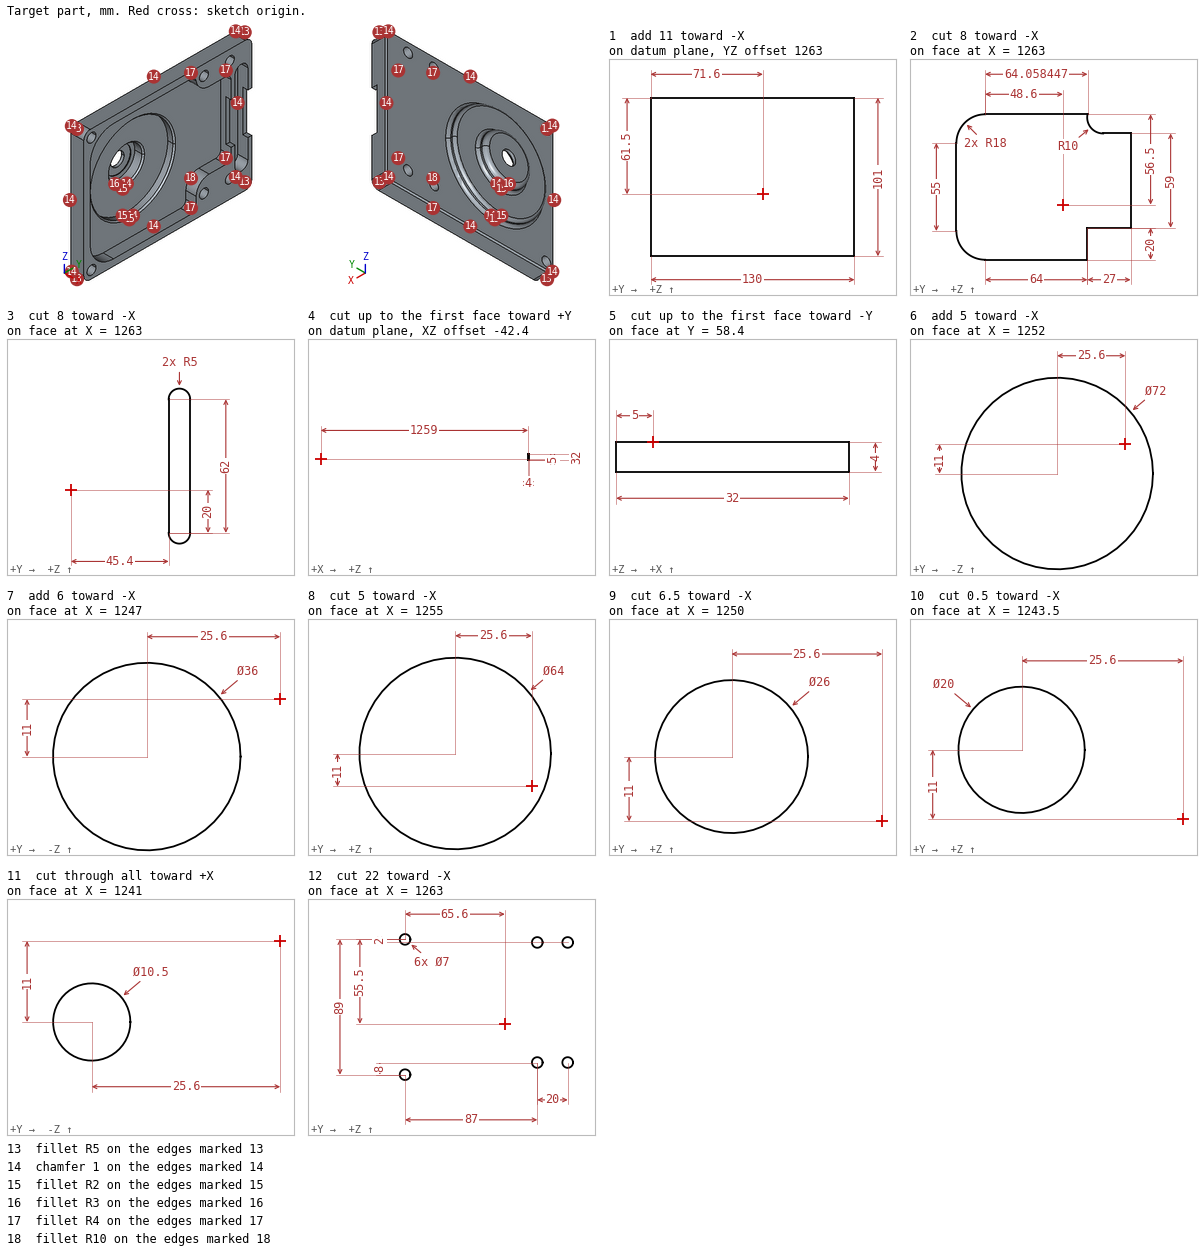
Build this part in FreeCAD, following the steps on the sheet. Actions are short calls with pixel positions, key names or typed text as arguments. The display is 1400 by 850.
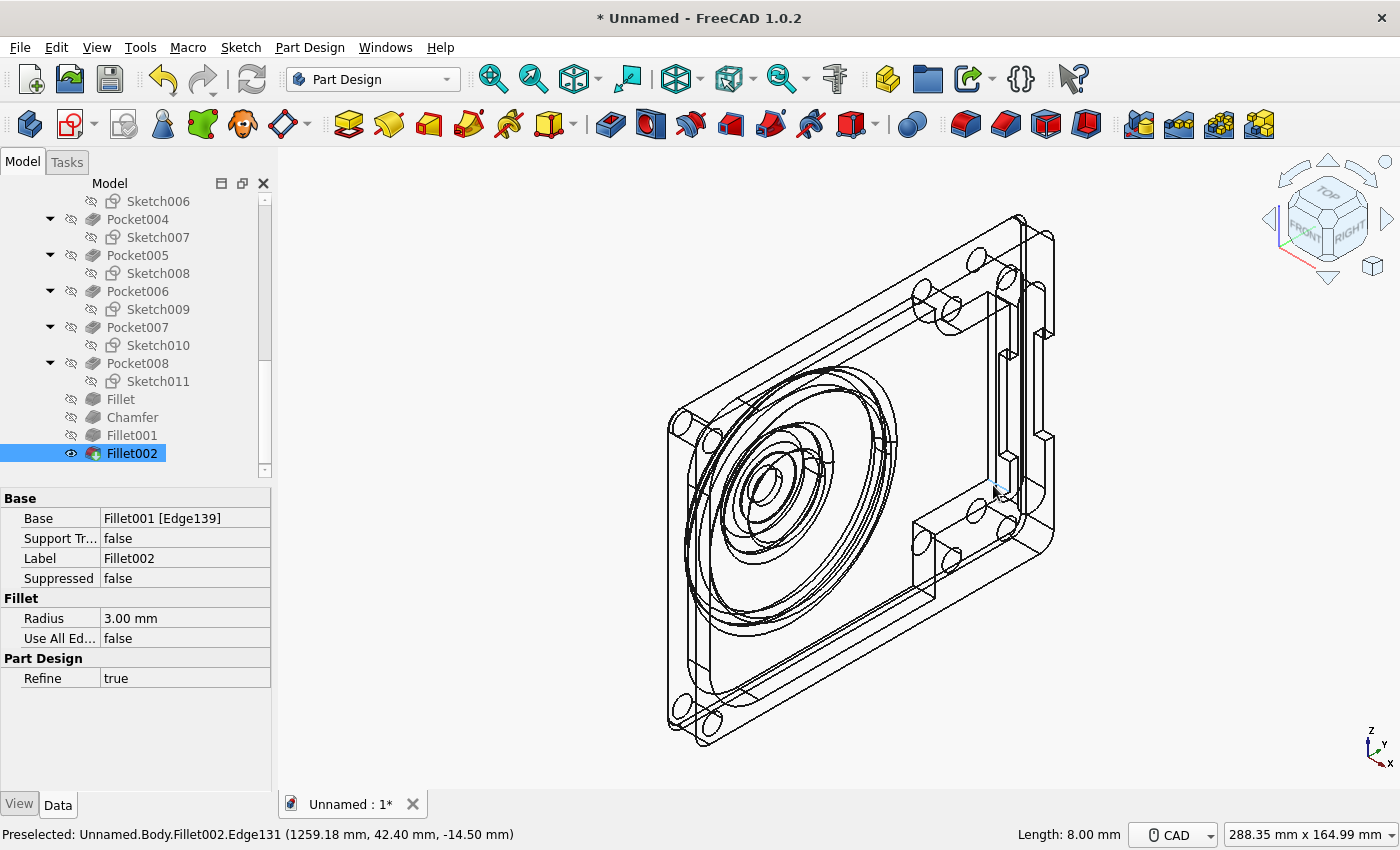
click(924, 591, ctrl)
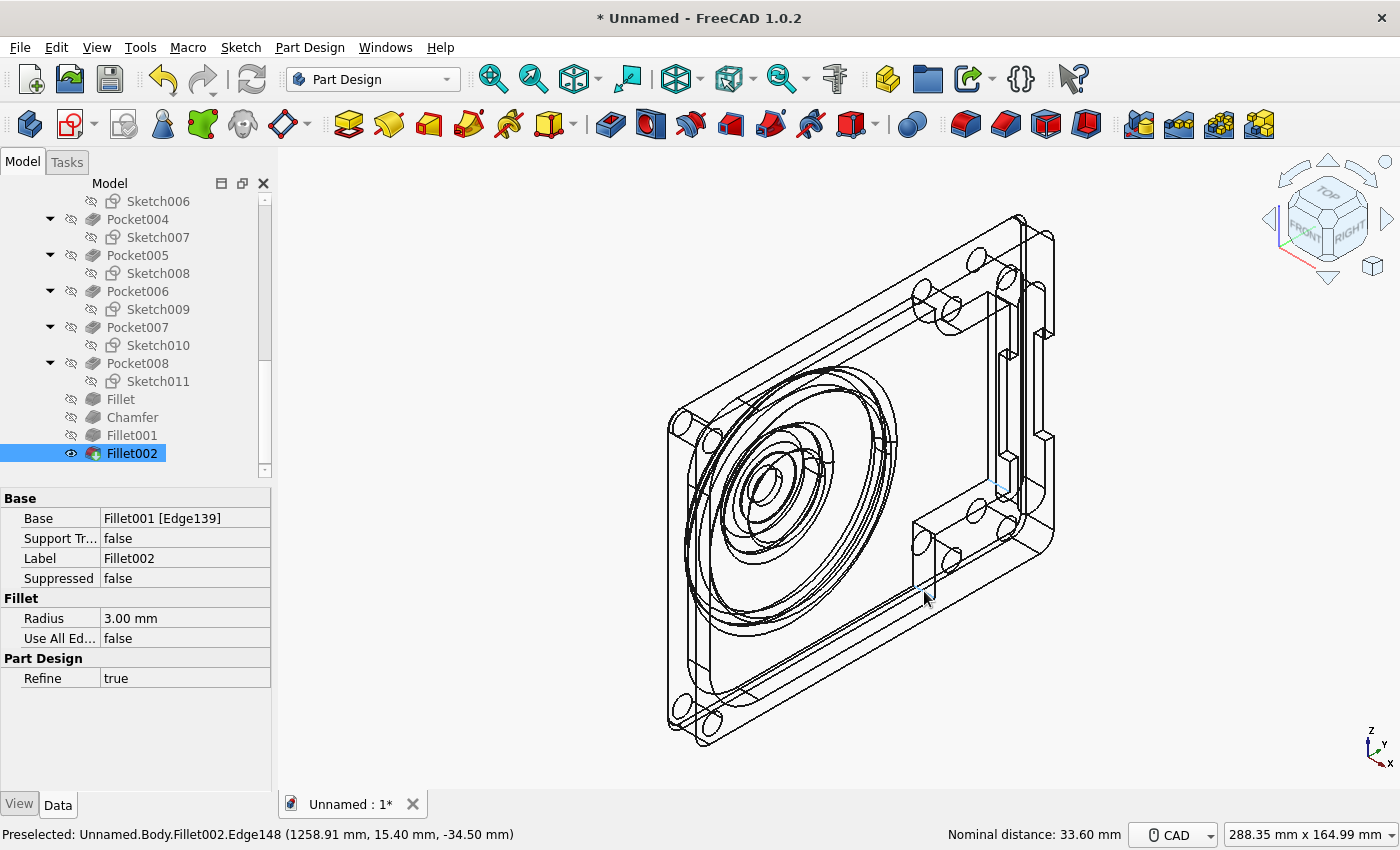
click(929, 304, ctrl)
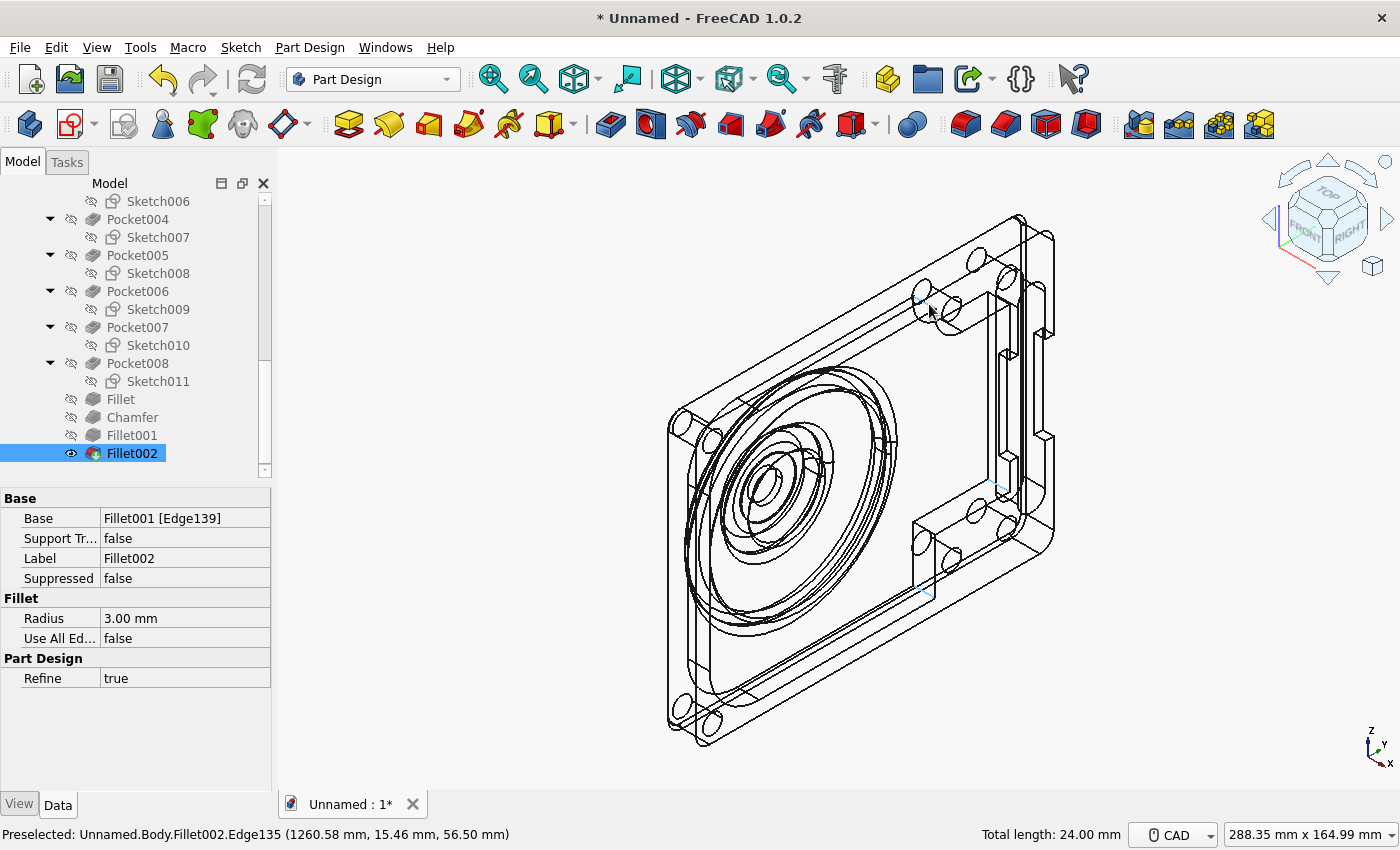
click(999, 297, ctrl)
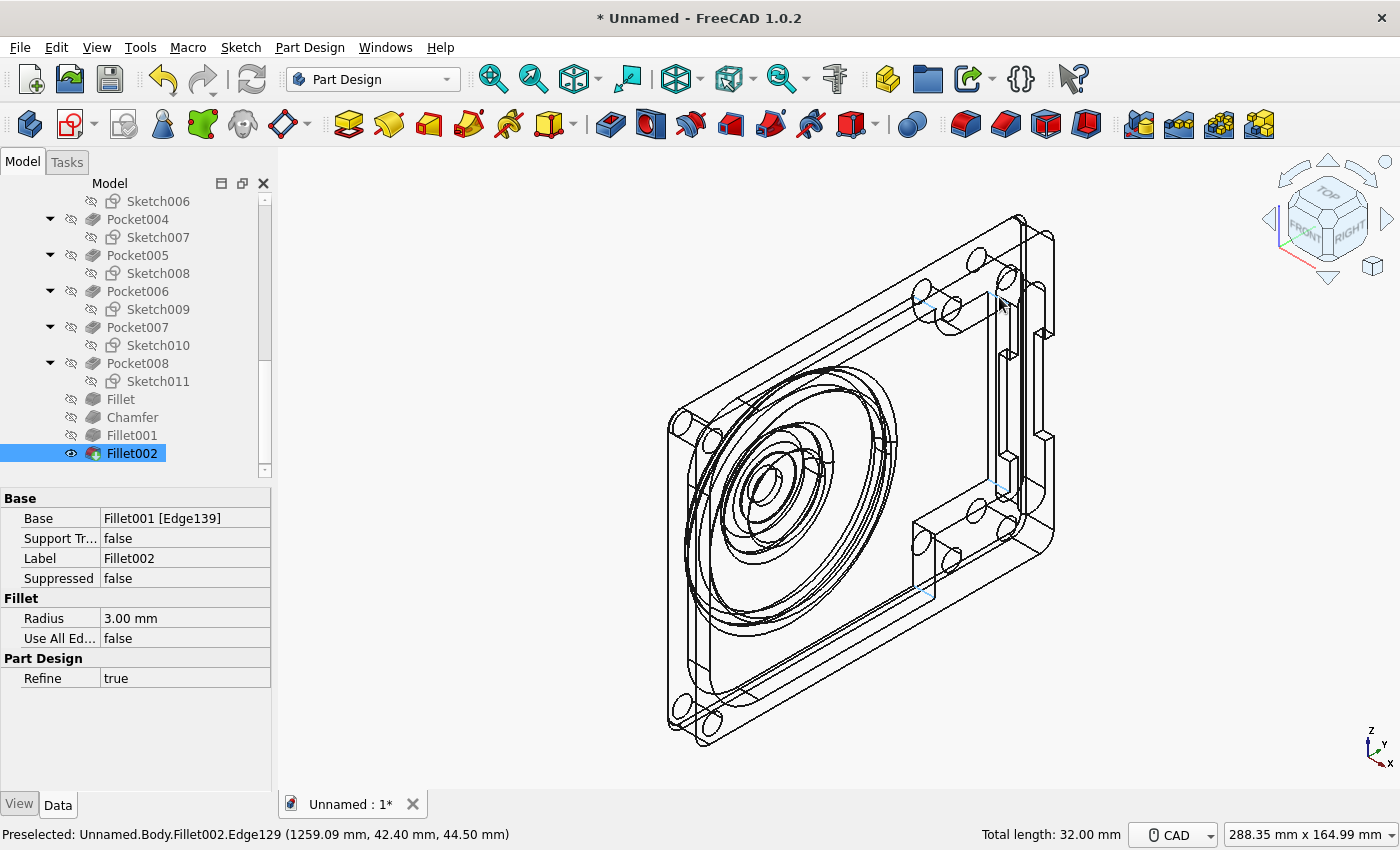
key(v)
key(1)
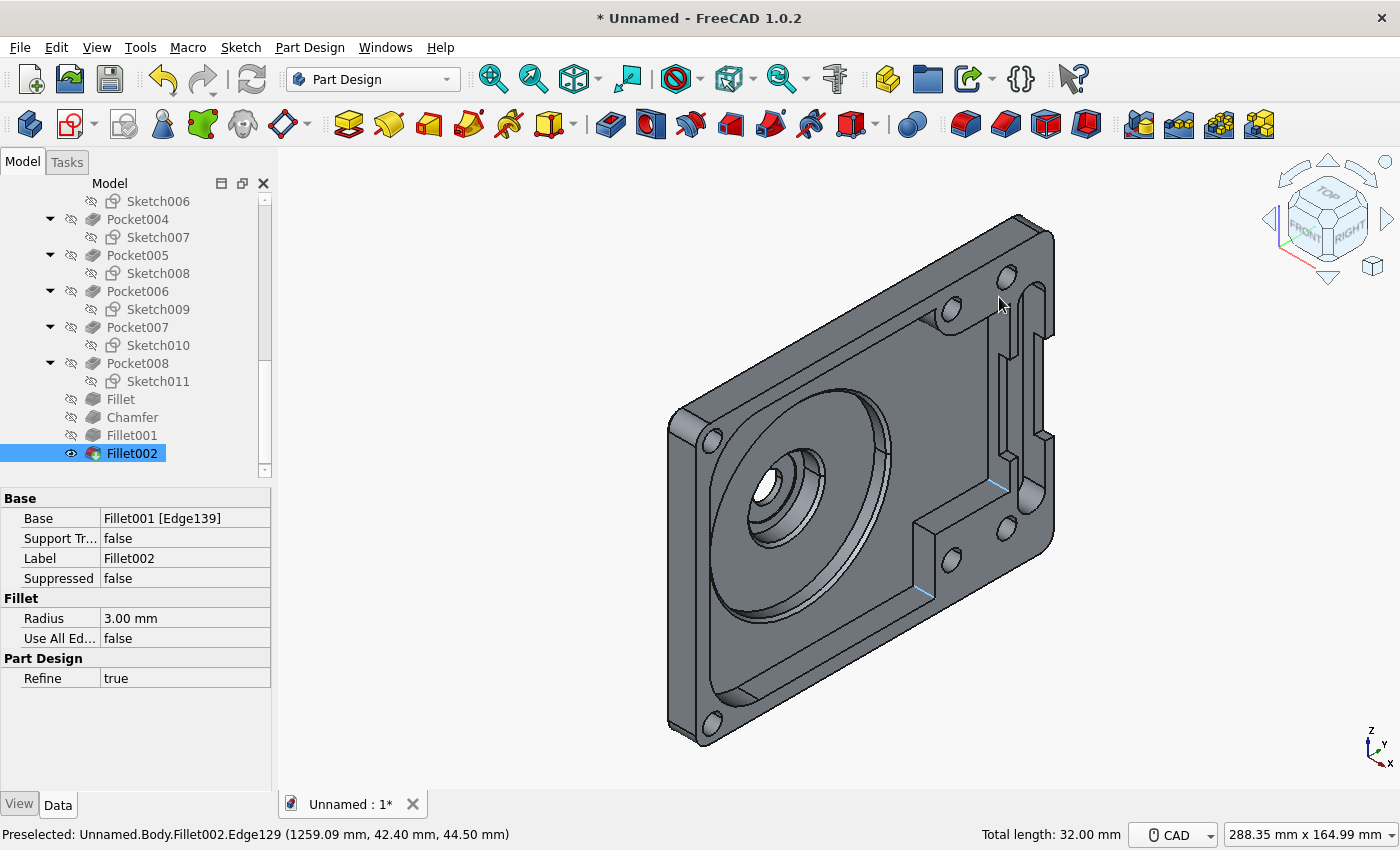
click(966, 124)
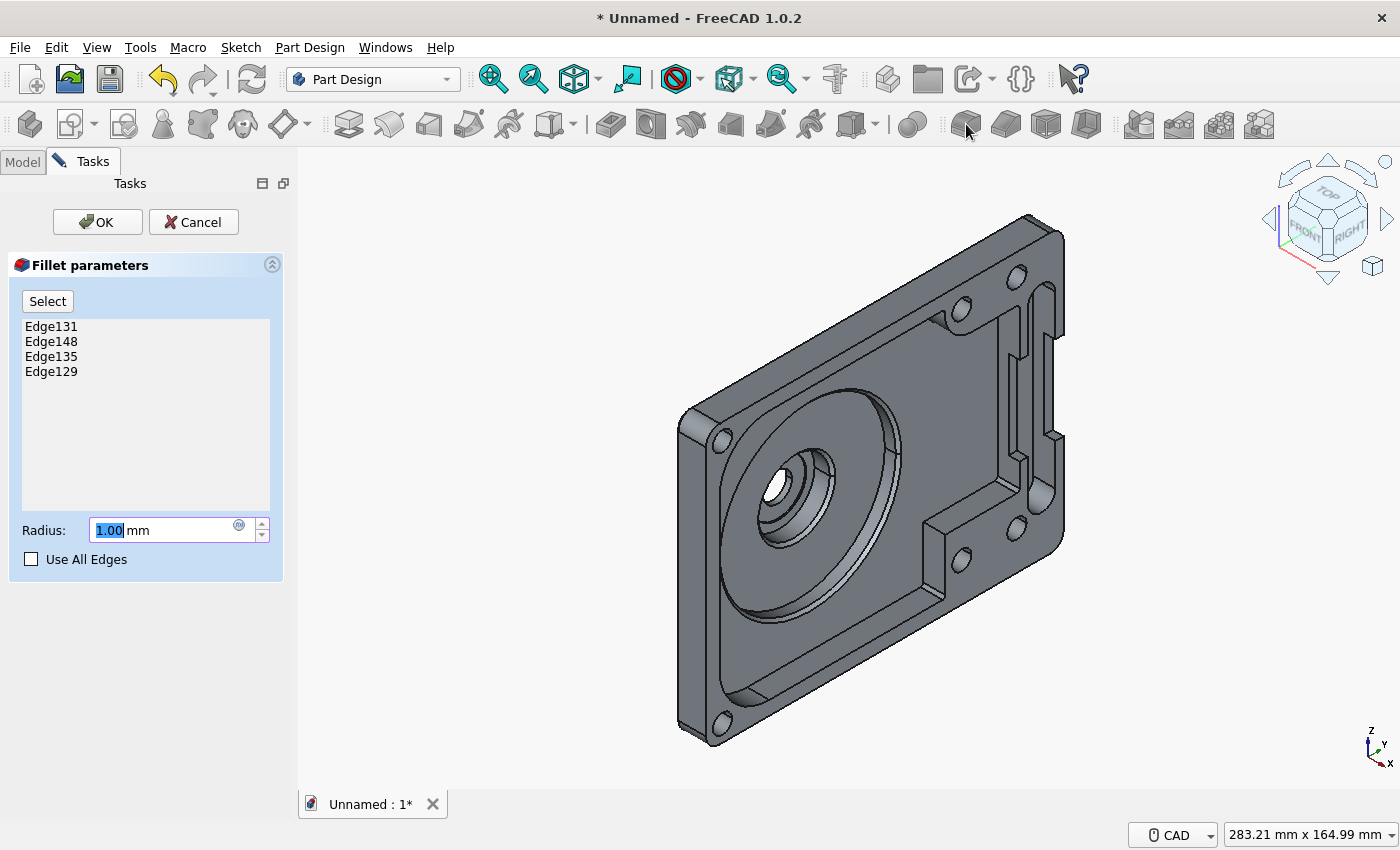
text(4)
key(Tab)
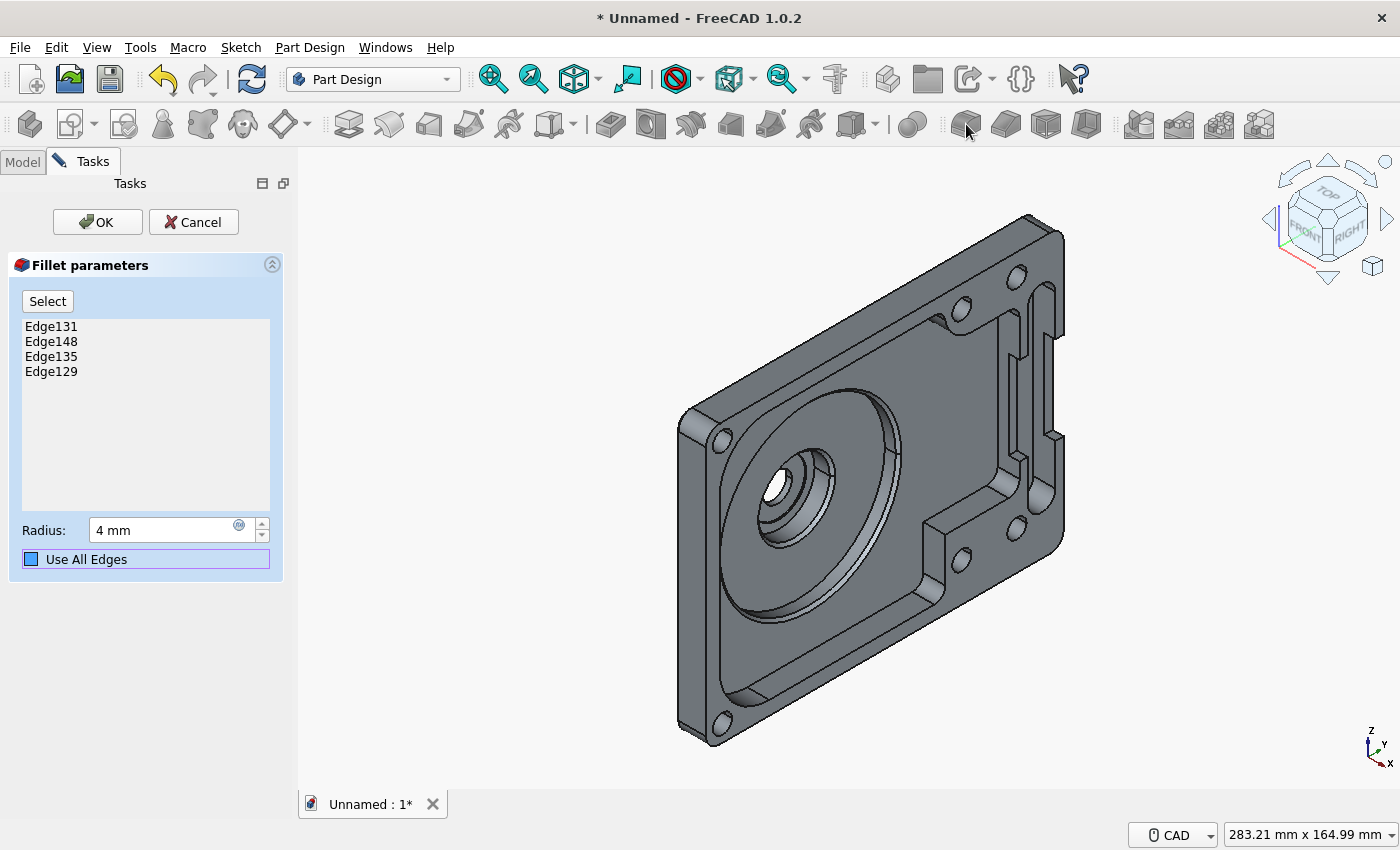
click(98, 222)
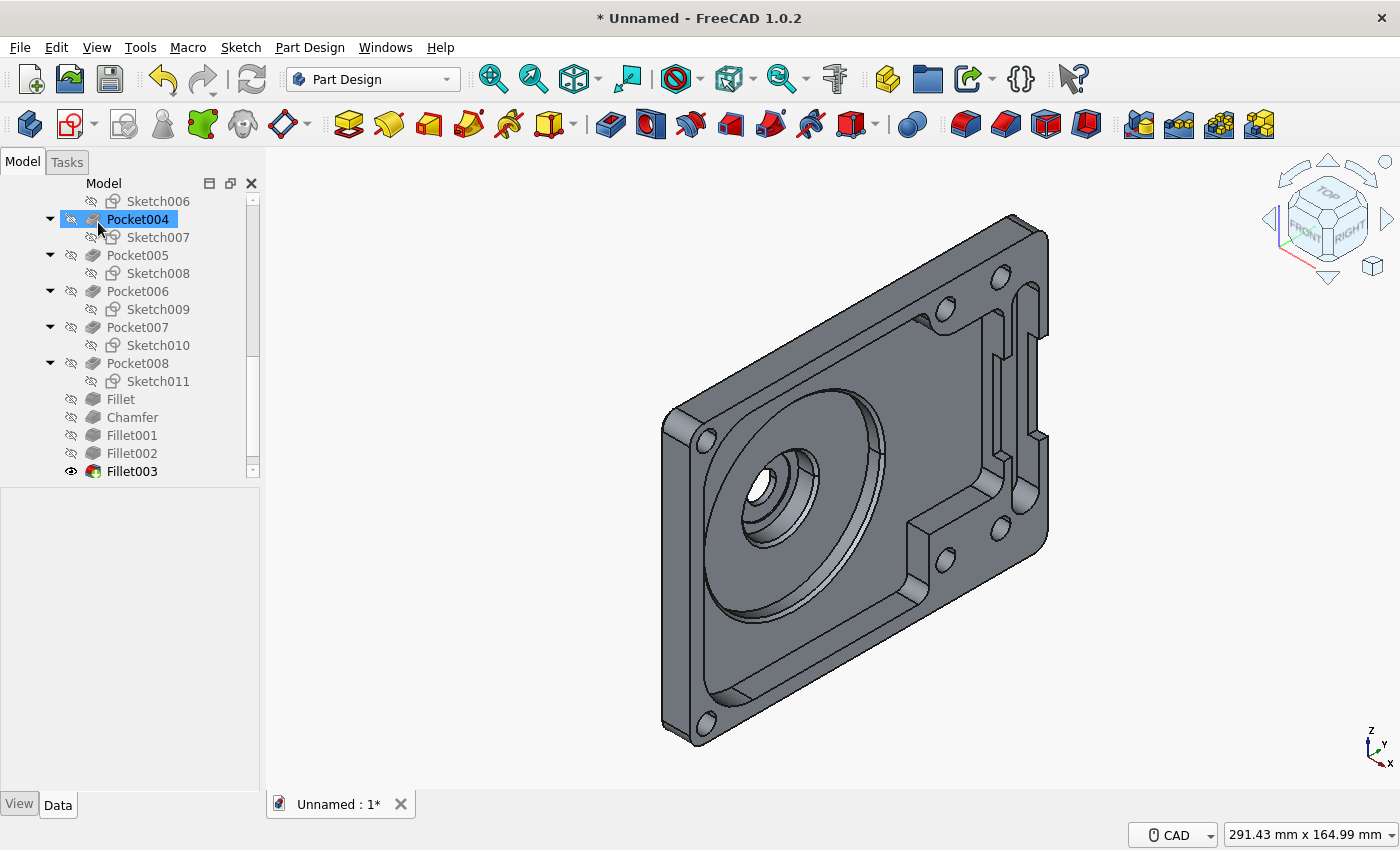
click(918, 527)